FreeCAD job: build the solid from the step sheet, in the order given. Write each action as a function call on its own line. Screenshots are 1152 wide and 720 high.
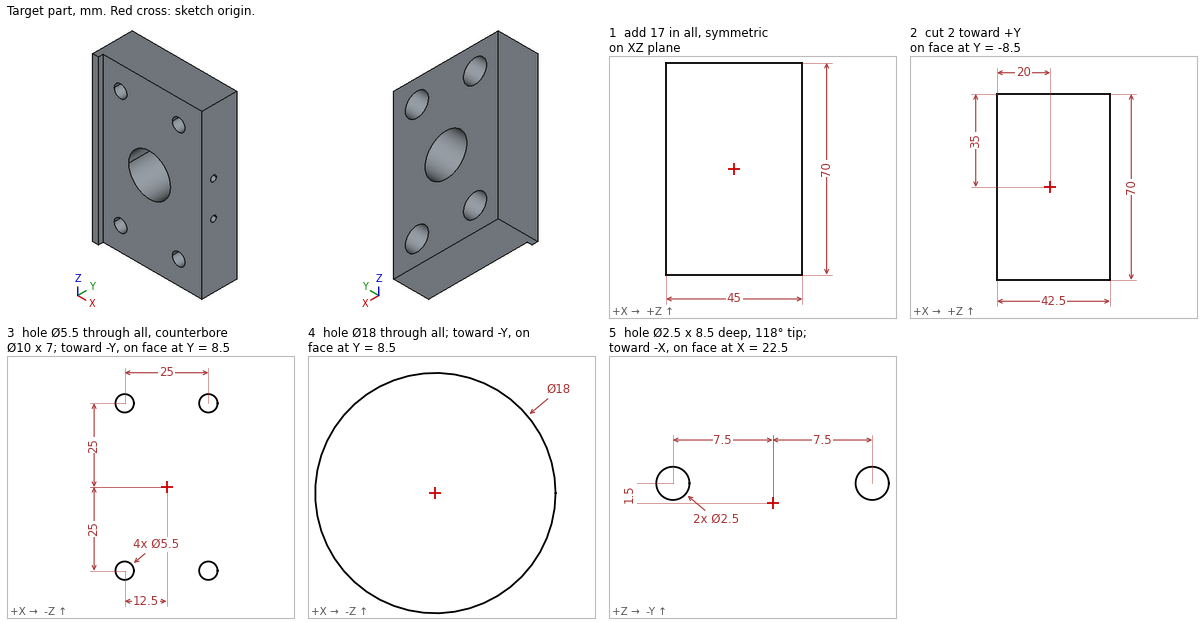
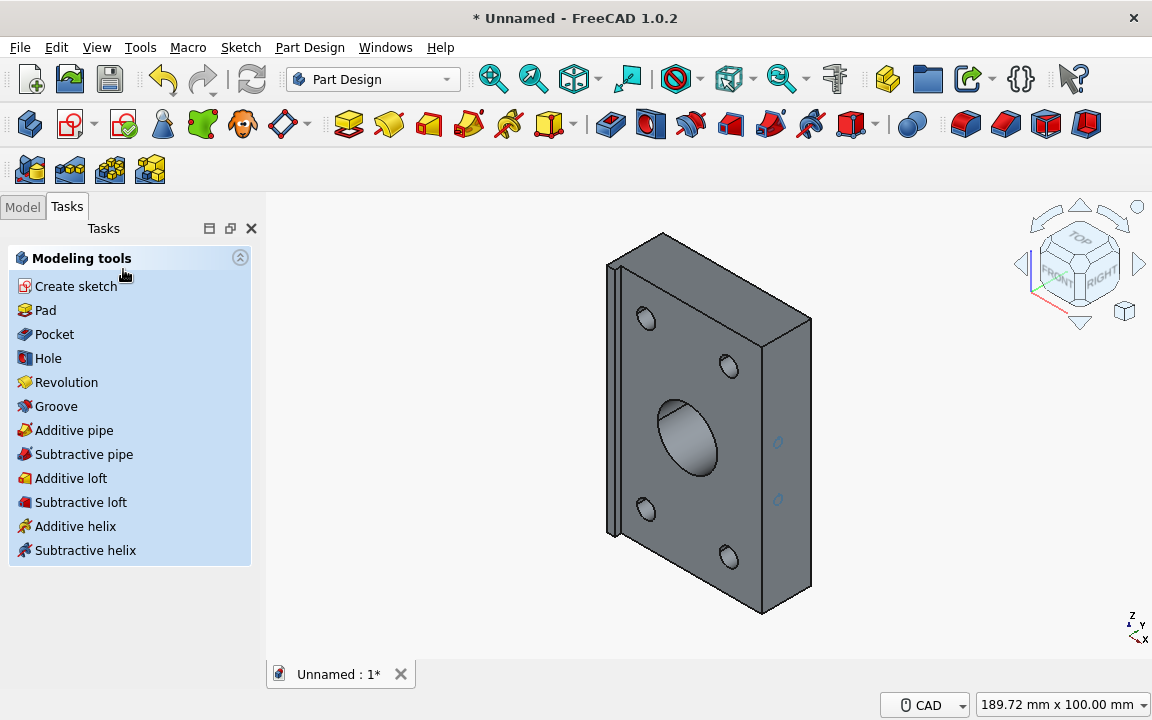
click(652, 124)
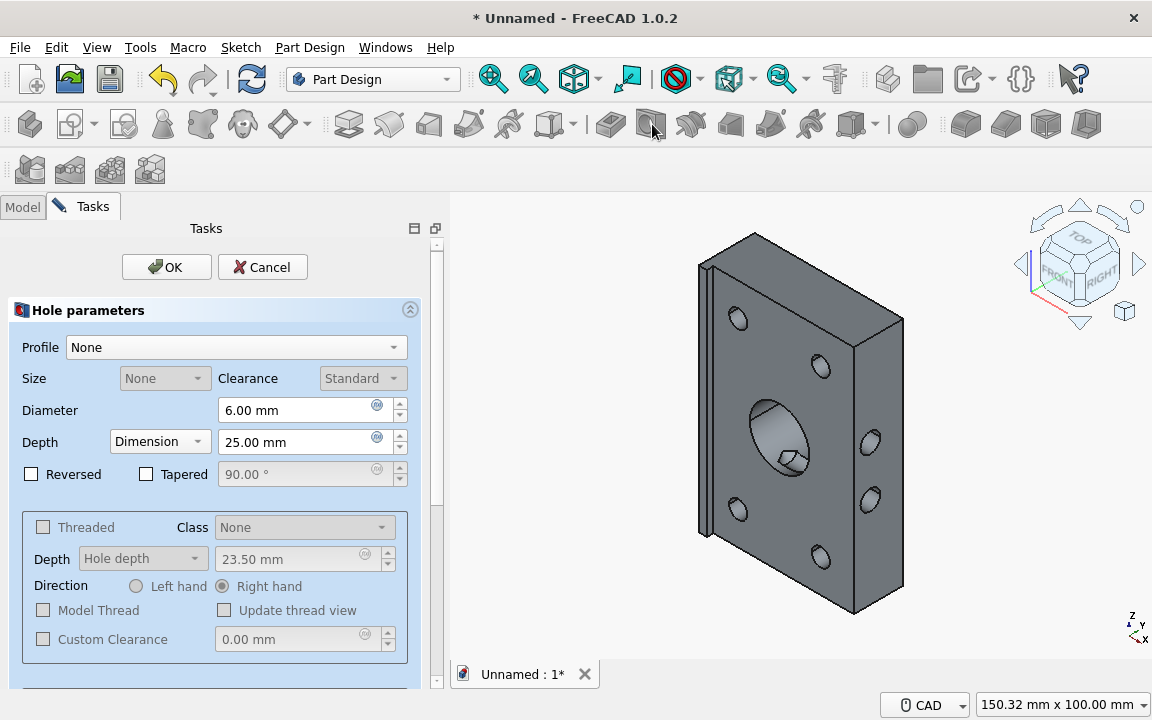
triple_click(305, 410)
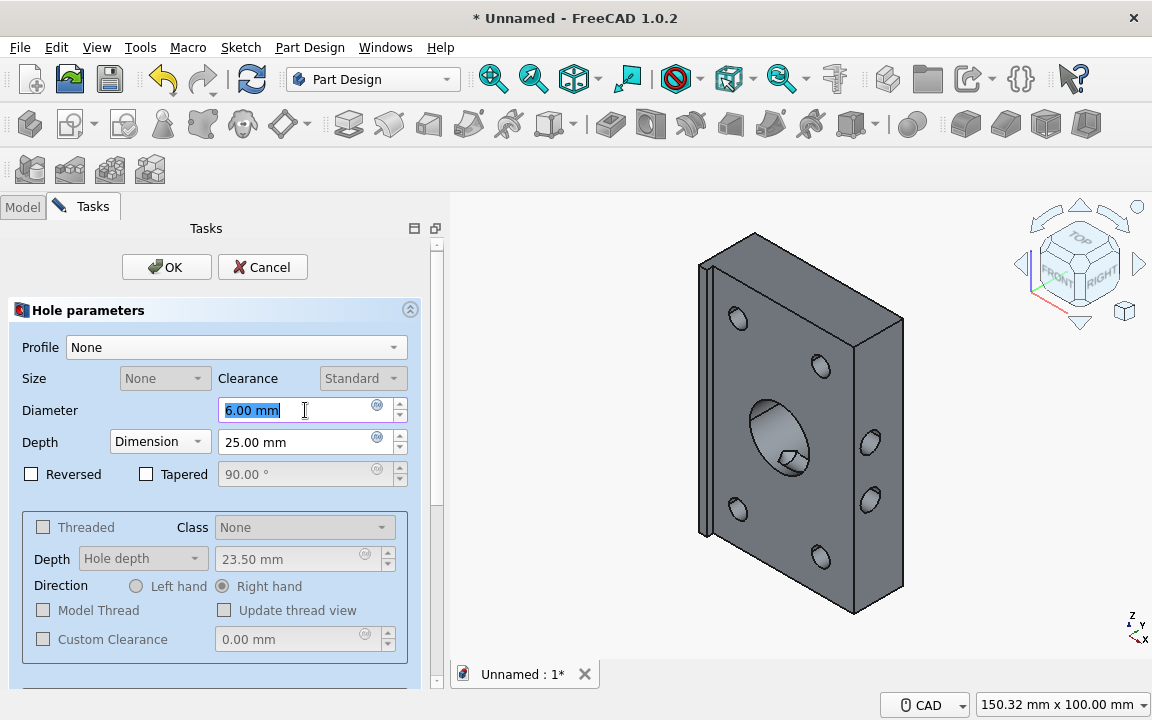
text(2.5)
key(Tab)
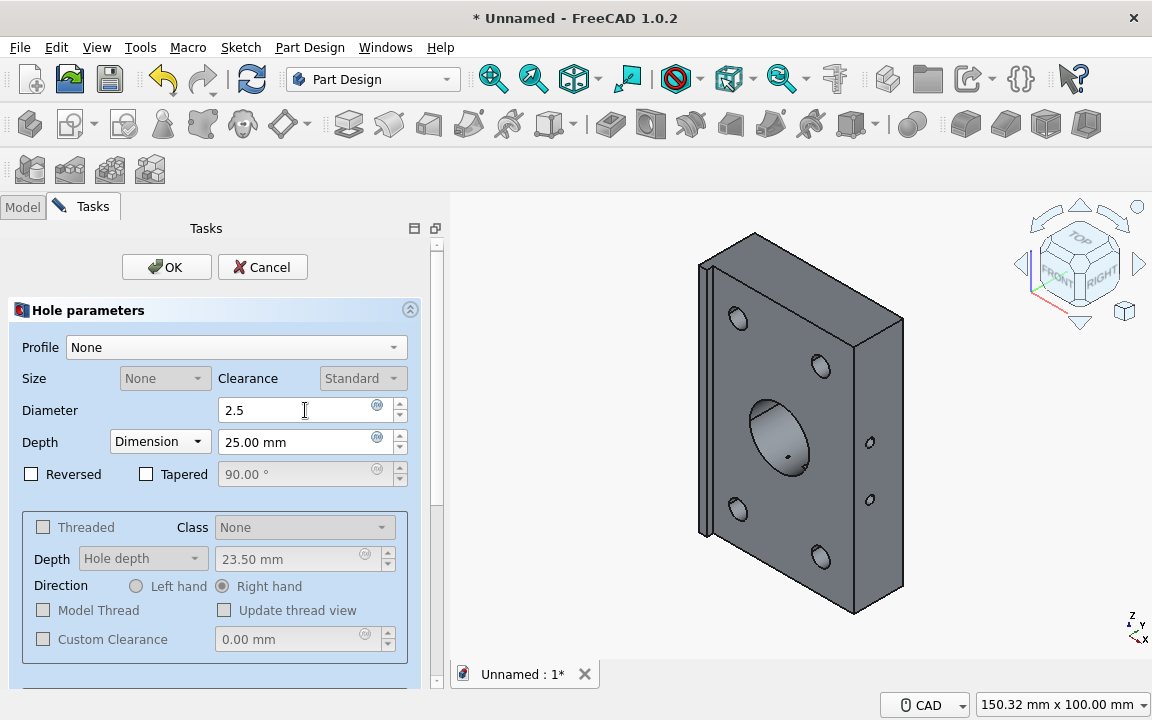
triple_click(305, 442)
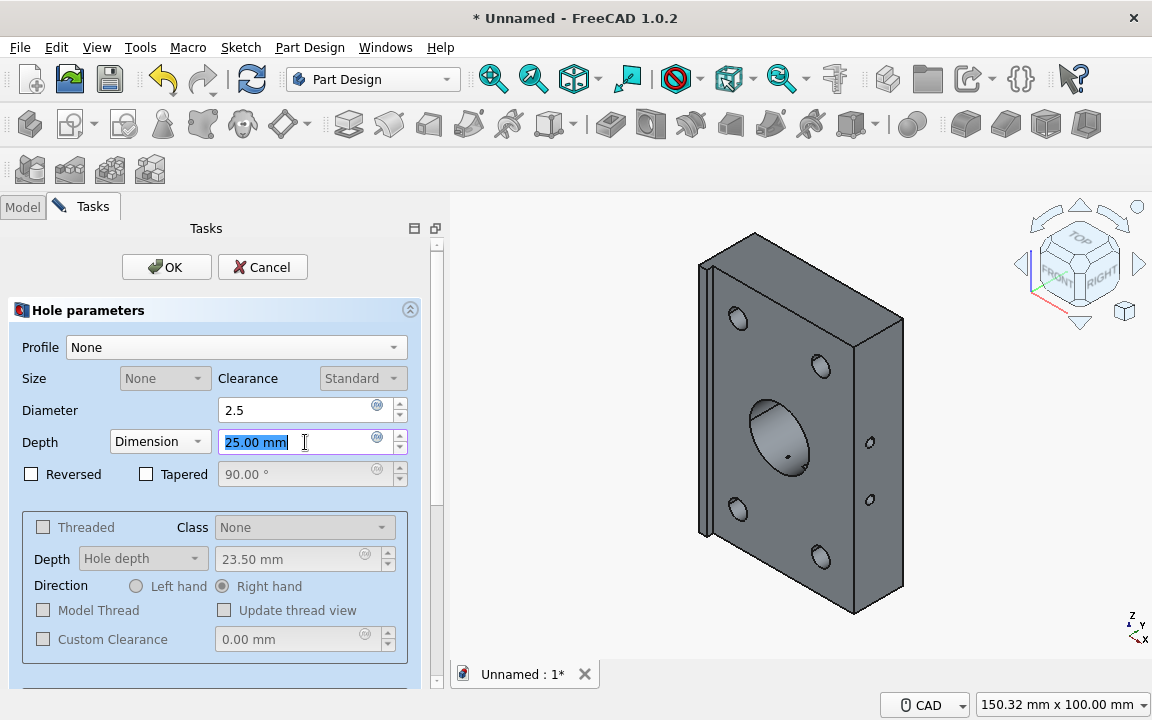
text(8.5)
key(Tab)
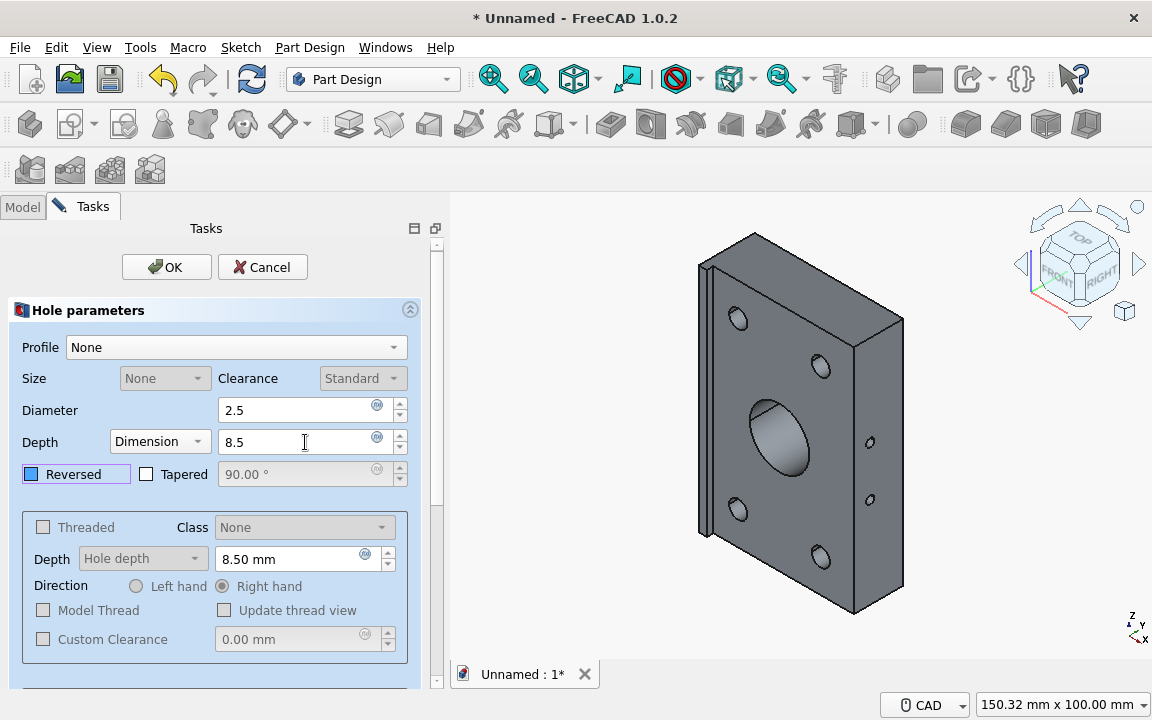
click(167, 267)